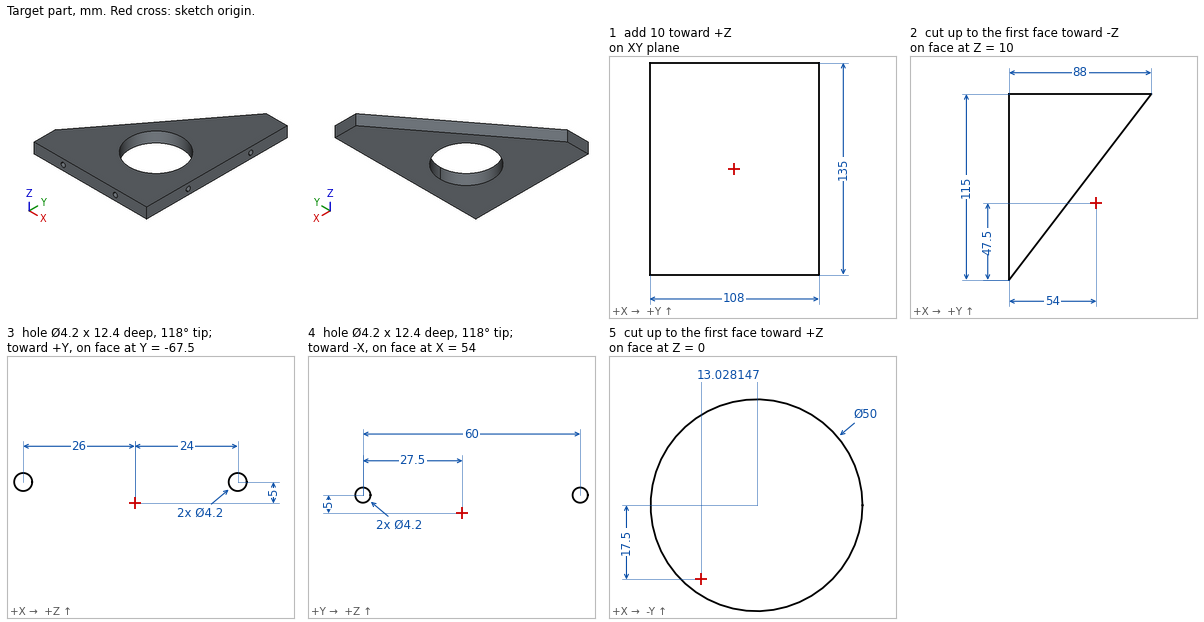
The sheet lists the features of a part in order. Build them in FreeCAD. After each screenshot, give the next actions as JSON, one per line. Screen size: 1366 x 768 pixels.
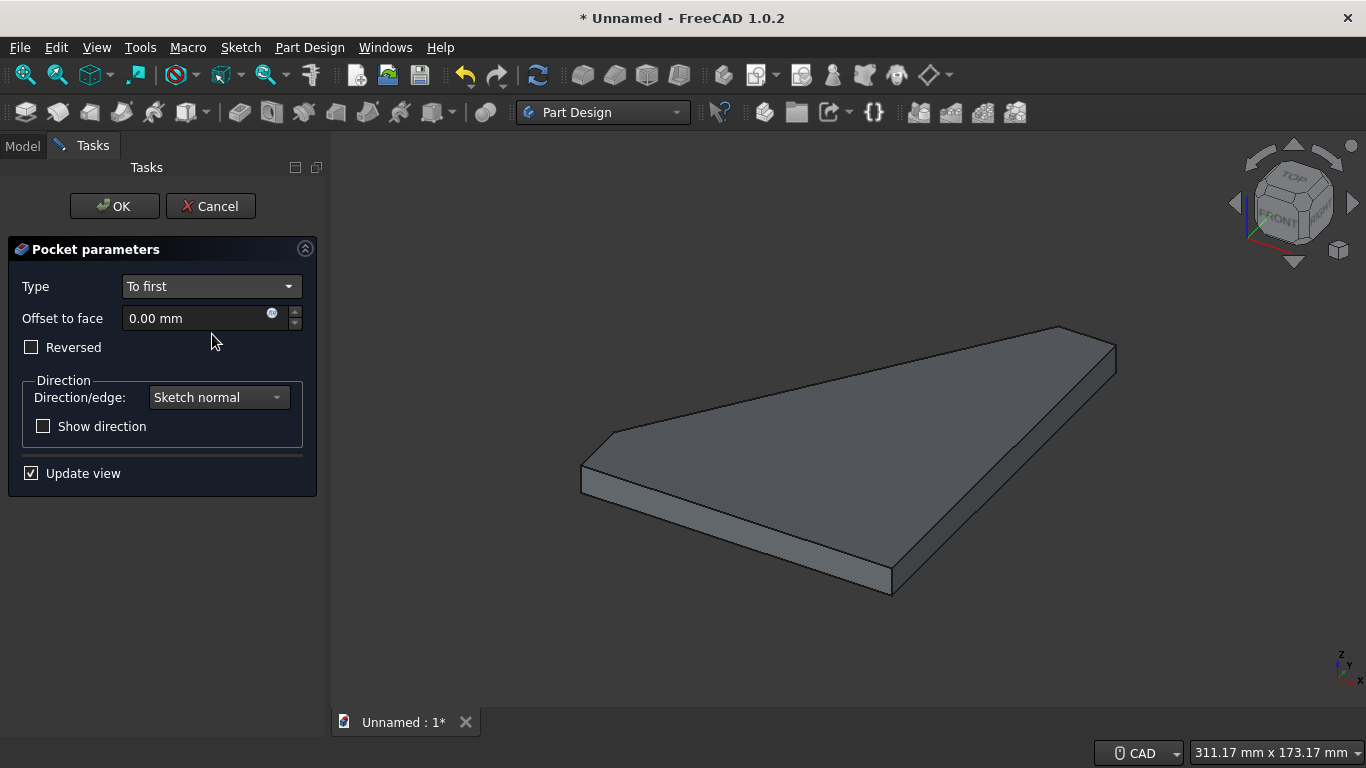
{"action": "left_click", "coordinate": [115, 206]}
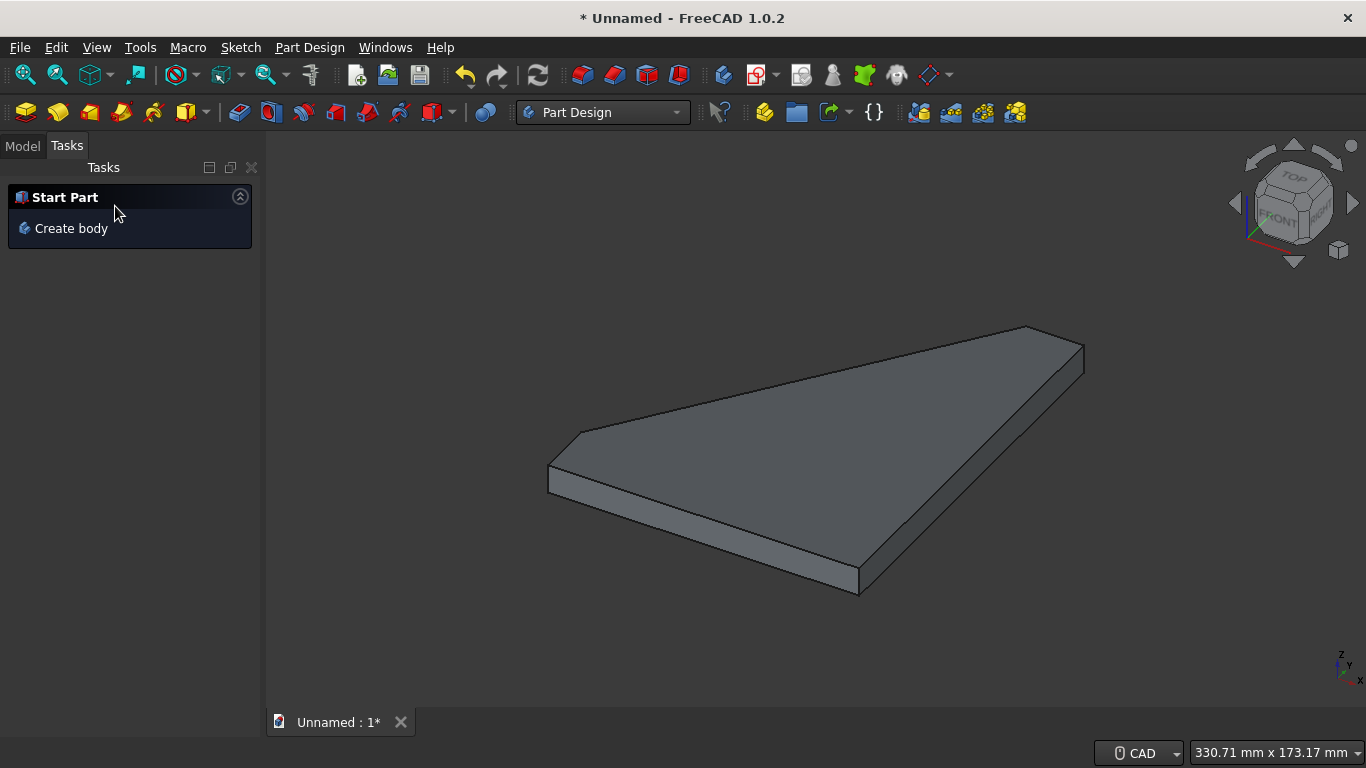
{"action": "left_click", "coordinate": [837, 574]}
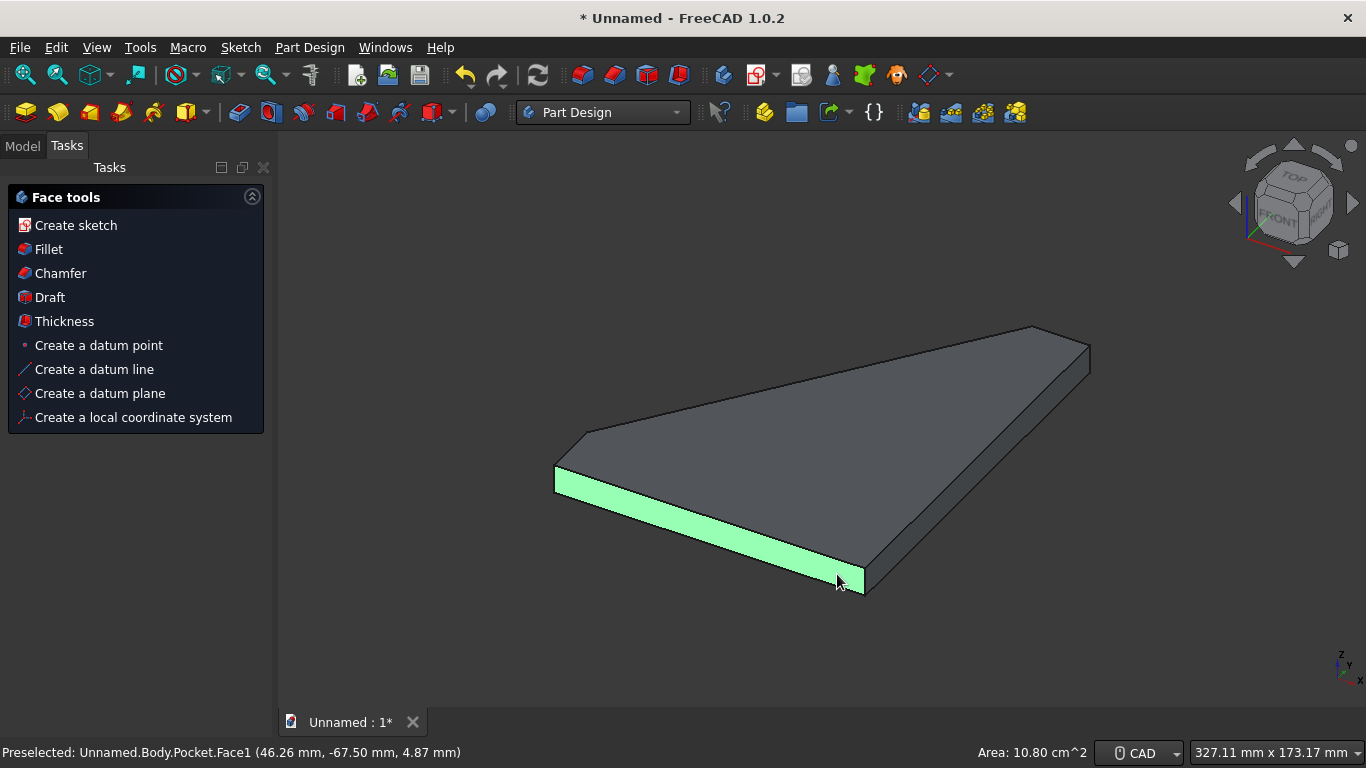
{"action": "left_click", "coordinate": [756, 76]}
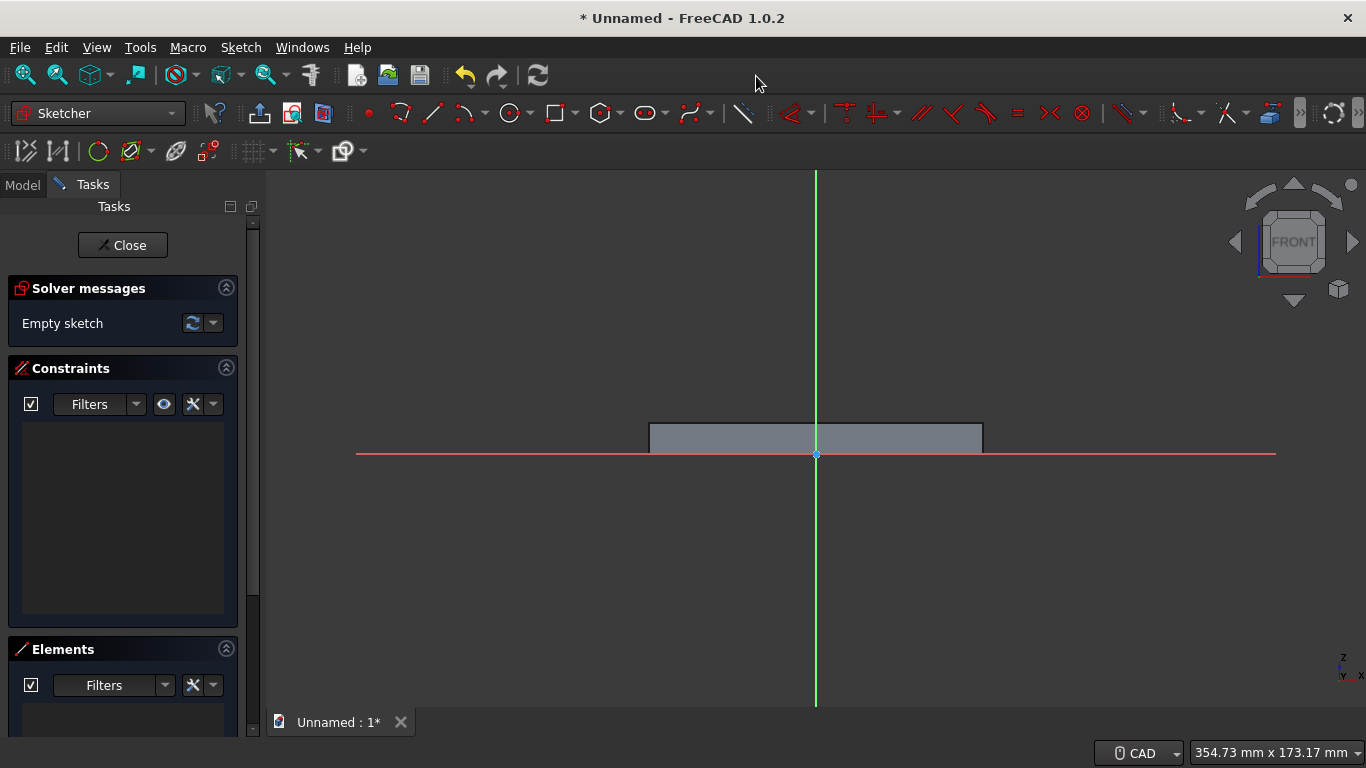
{"action": "scroll", "coordinate": [834, 444], "scroll_direction": "up", "scroll_amount": 7}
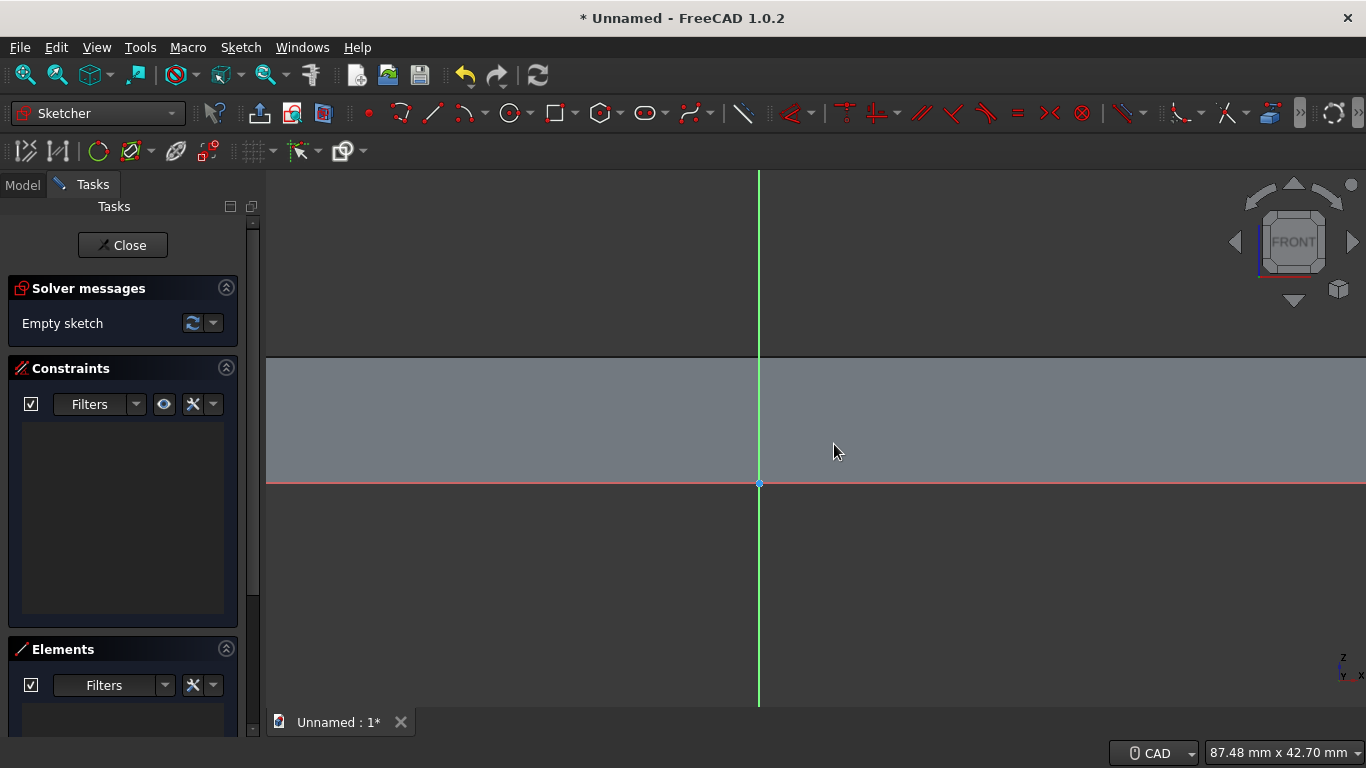
{"action": "key", "text": "g c"}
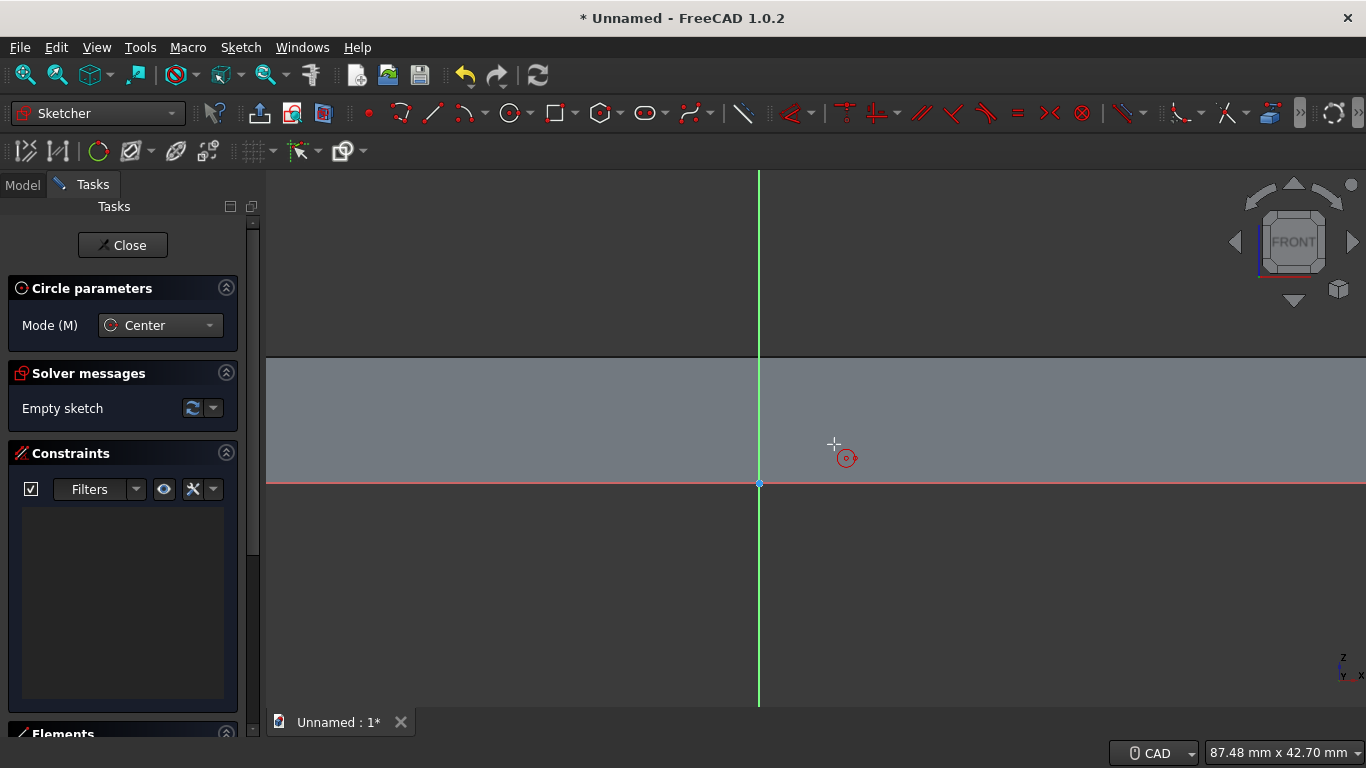
{"action": "left_click", "coordinate": [1061, 420]}
{"action": "mouse_move", "coordinate": [1080, 401]}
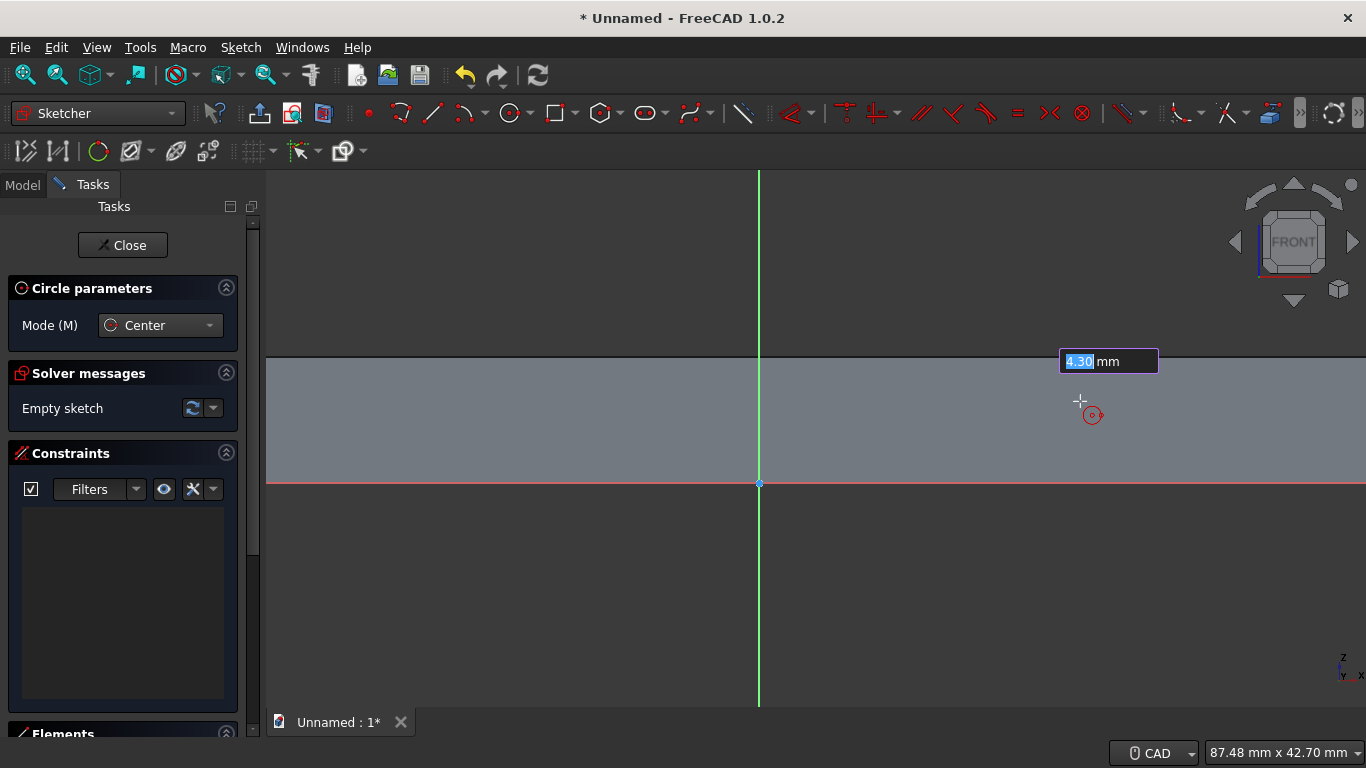
{"action": "type", "text": "4.2"}
{"action": "key", "text": "Return"}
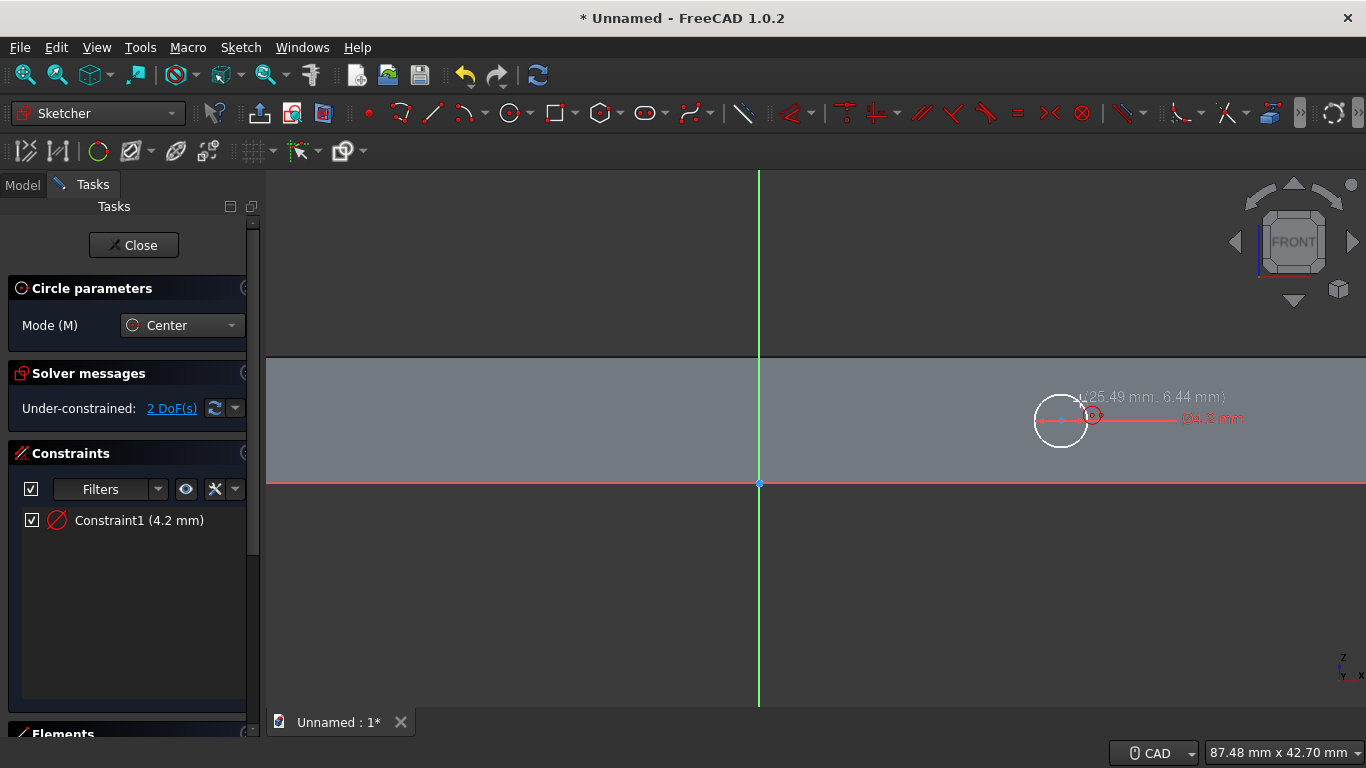
{"action": "left_click", "coordinate": [432, 420]}
{"action": "mouse_move", "coordinate": [451, 401]}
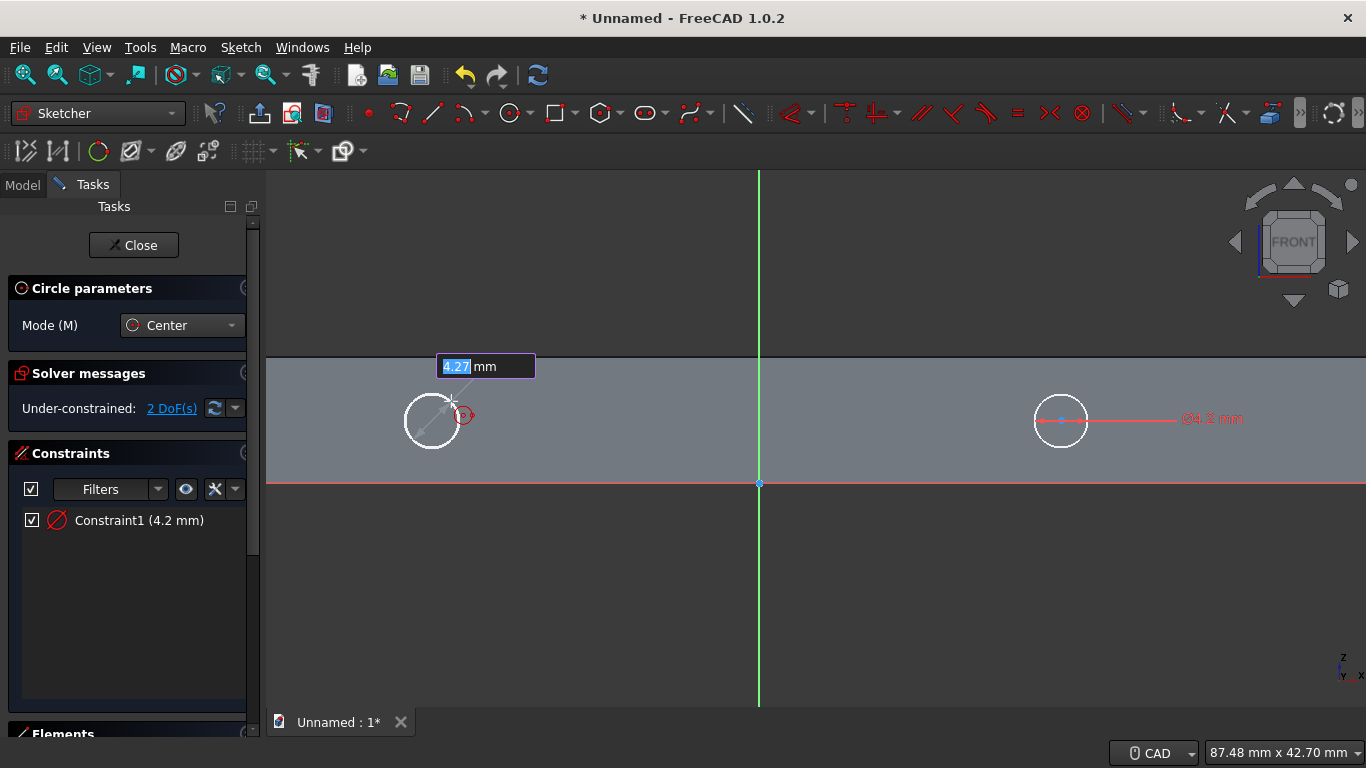
{"action": "type", "text": "4.2"}
{"action": "key", "text": "Return"}
{"action": "key", "text": "Escape"}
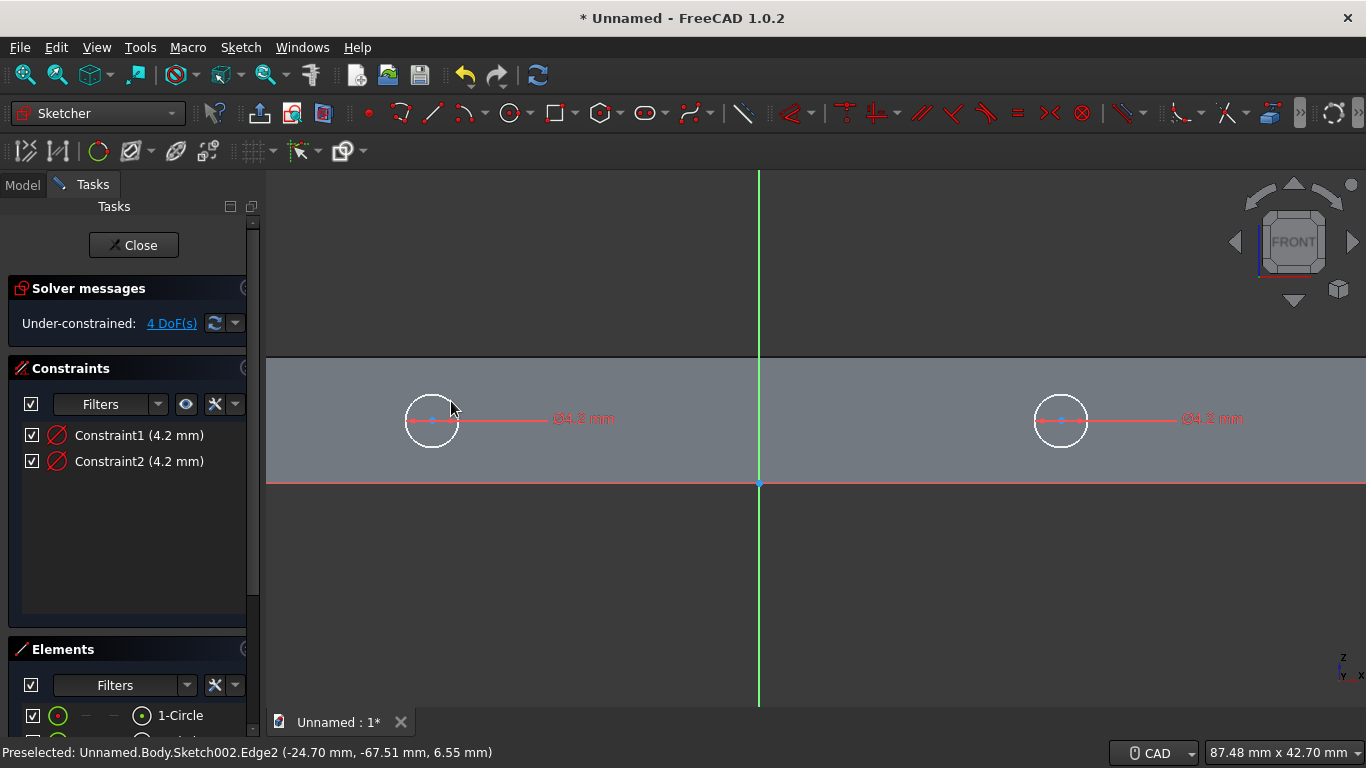
{"action": "left_click", "coordinate": [1061, 421]}